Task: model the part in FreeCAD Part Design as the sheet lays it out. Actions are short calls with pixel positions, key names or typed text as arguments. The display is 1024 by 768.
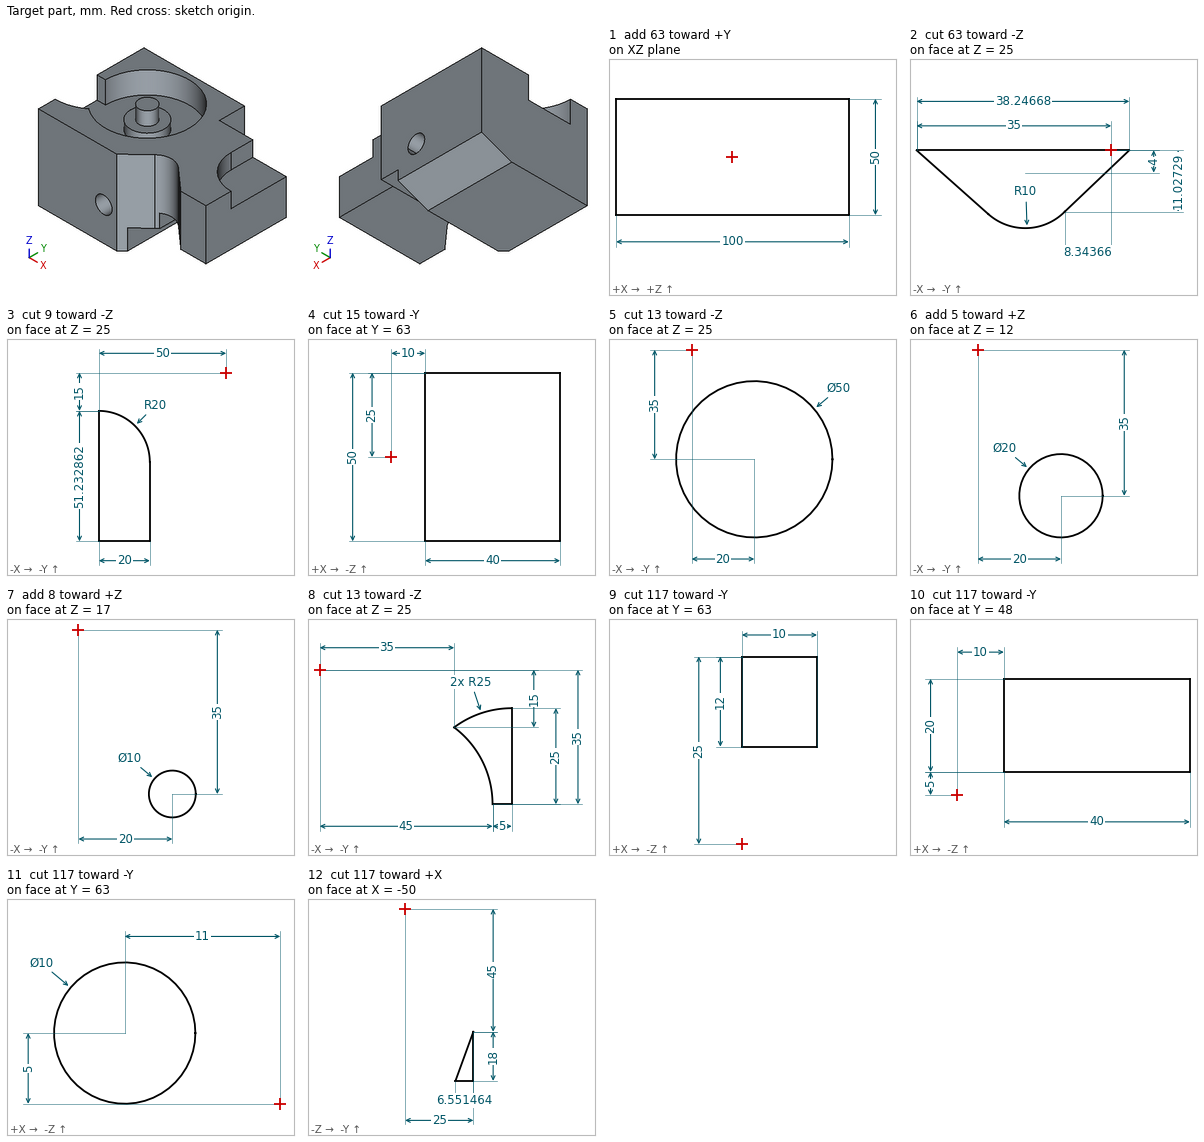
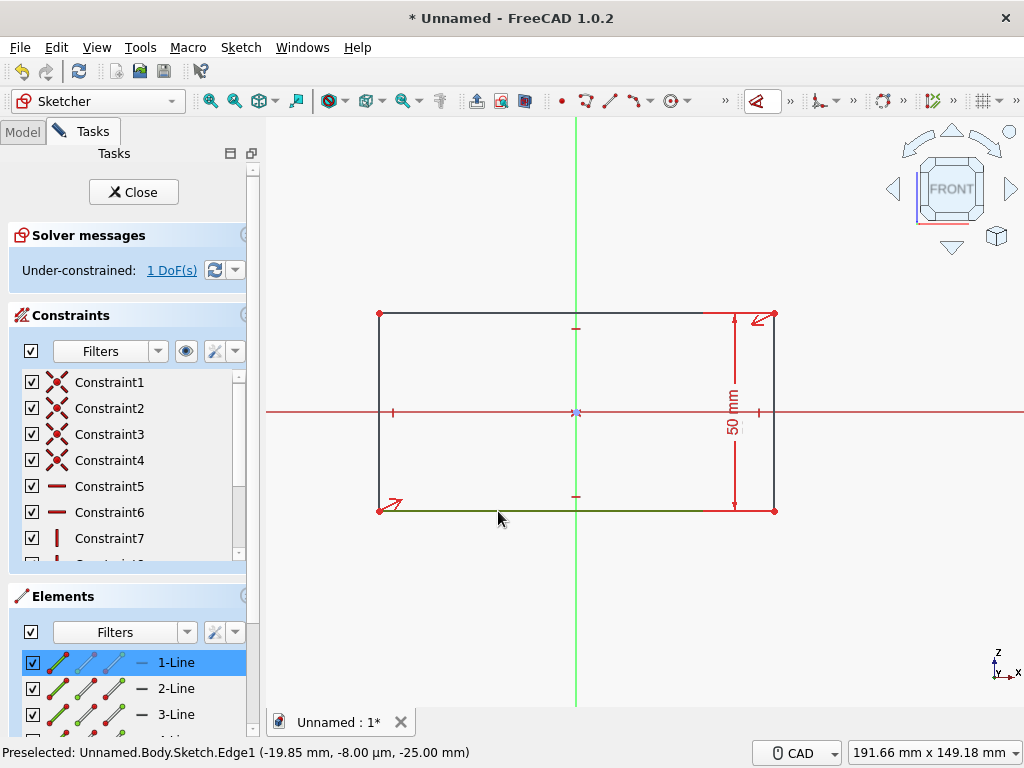
click(776, 102)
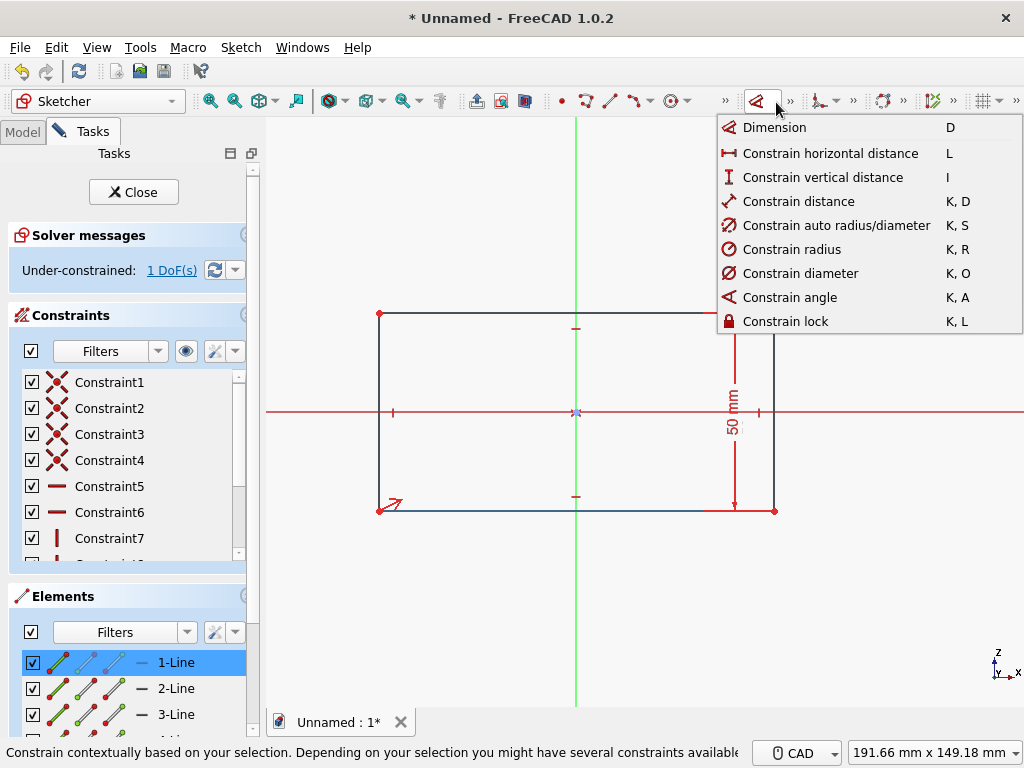
click(870, 153)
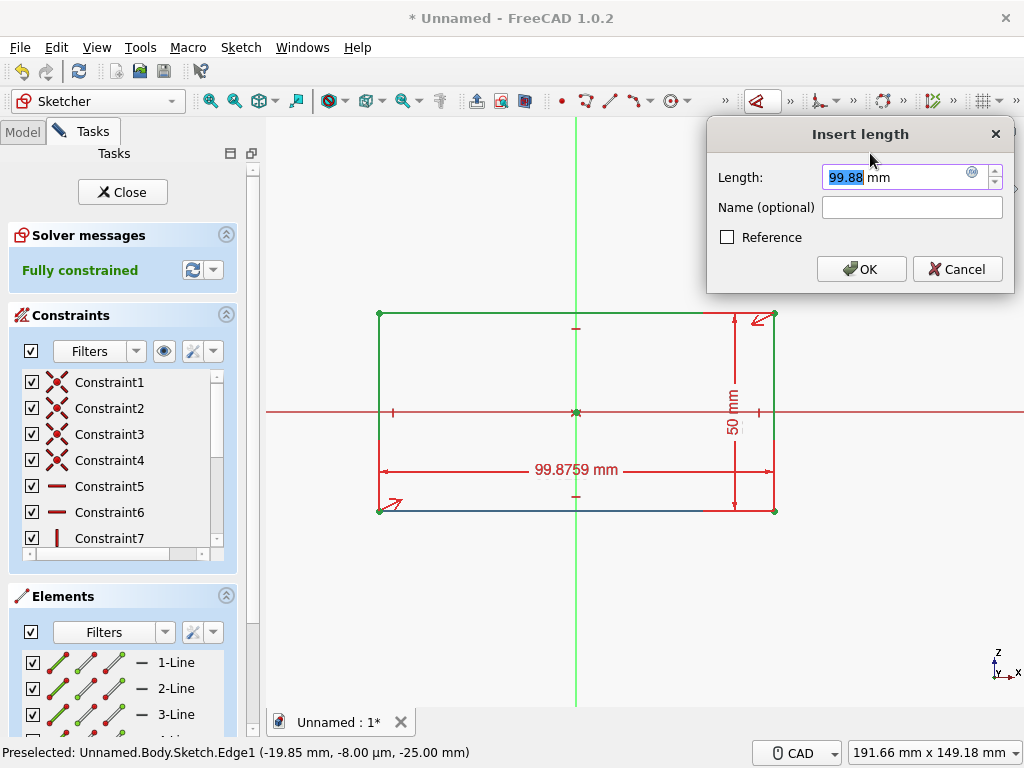
text(100)
key(Return)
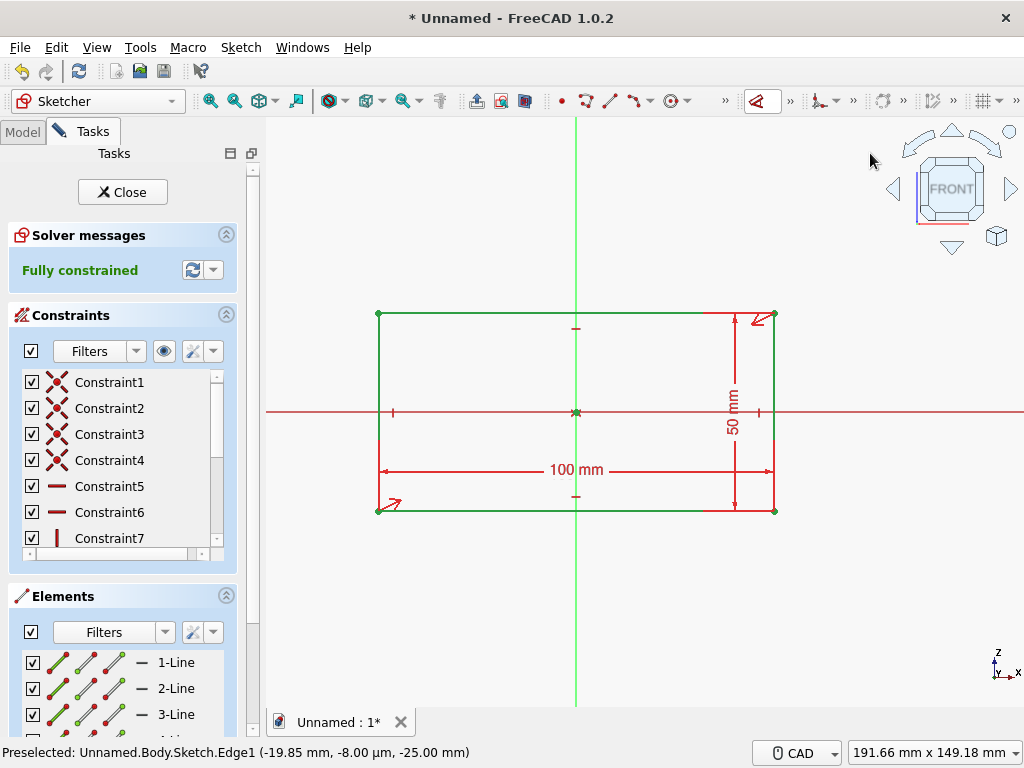
click(123, 192)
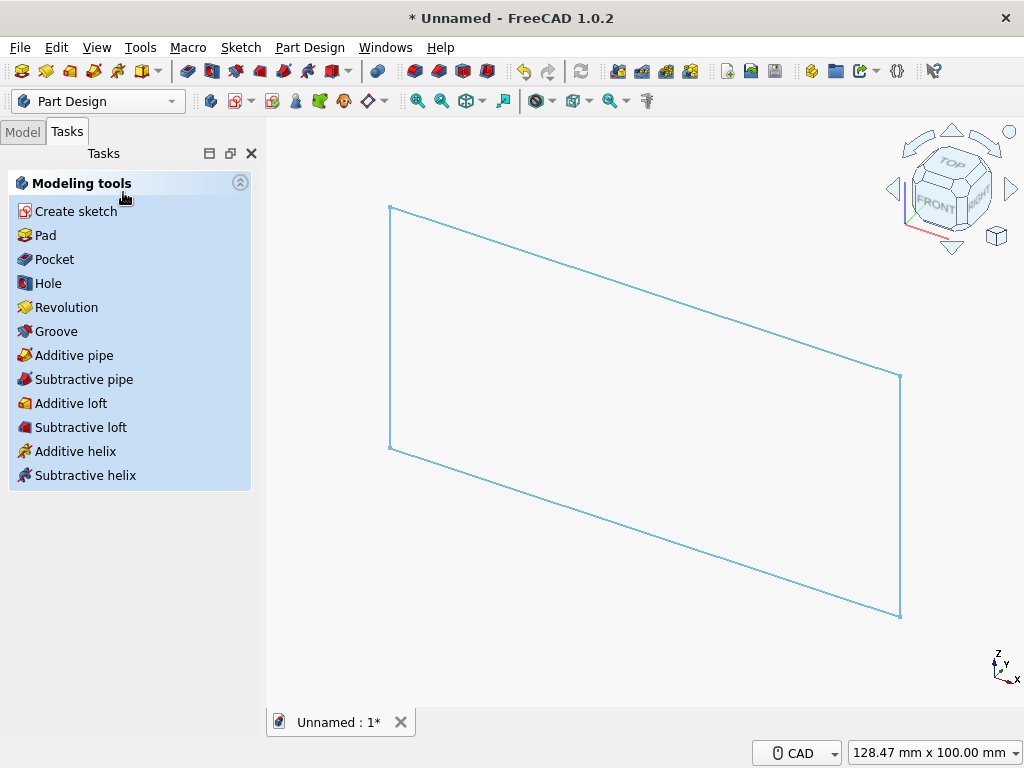
click(22, 72)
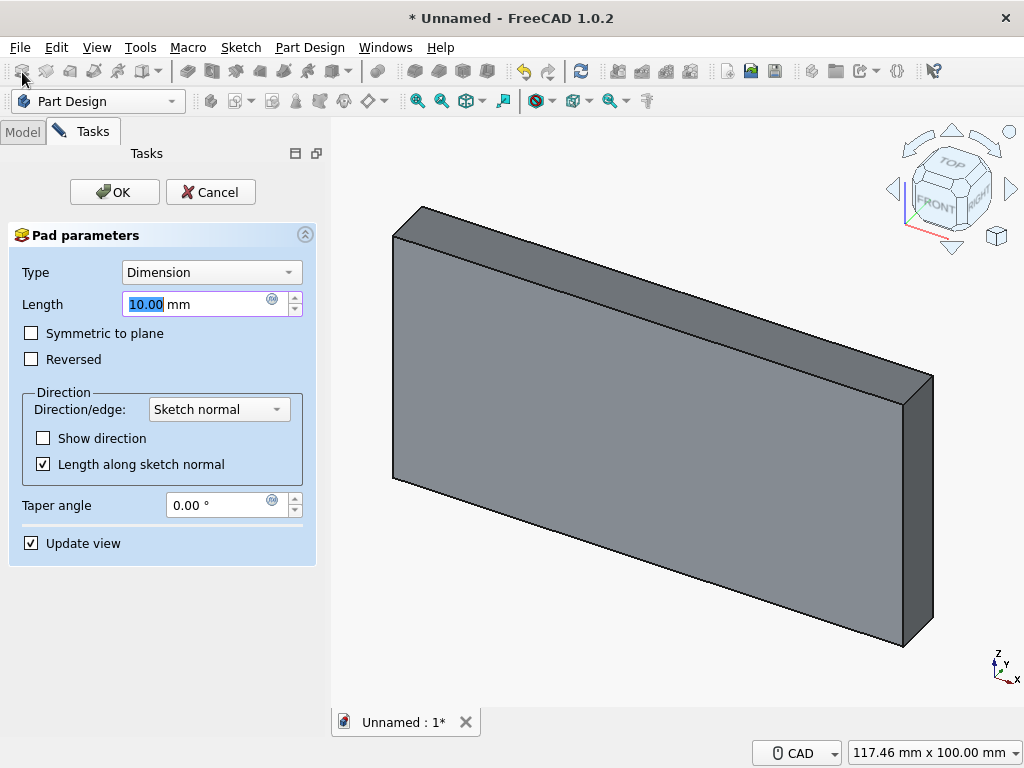
text(63)
key(Tab)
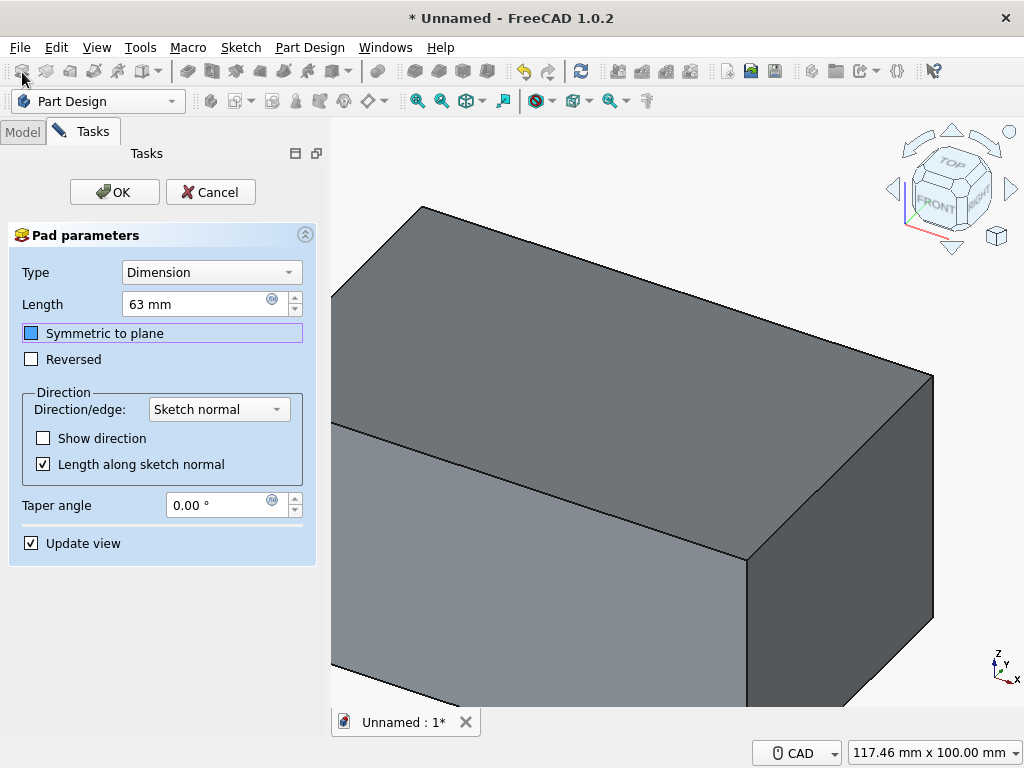
click(30, 359)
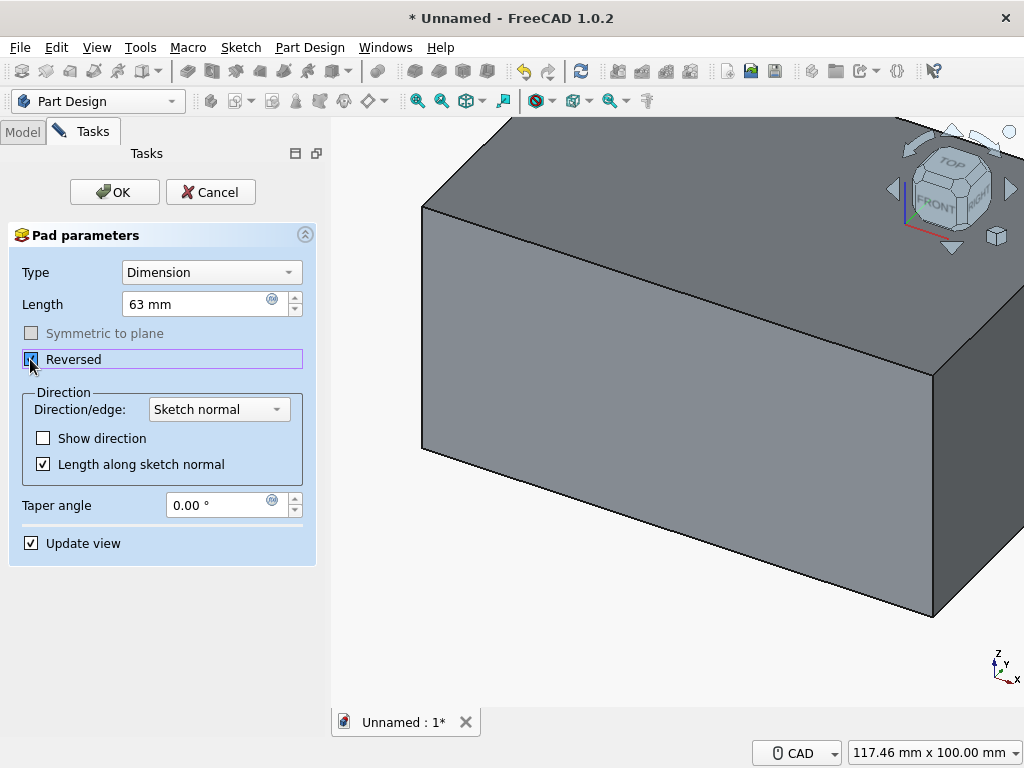
click(115, 192)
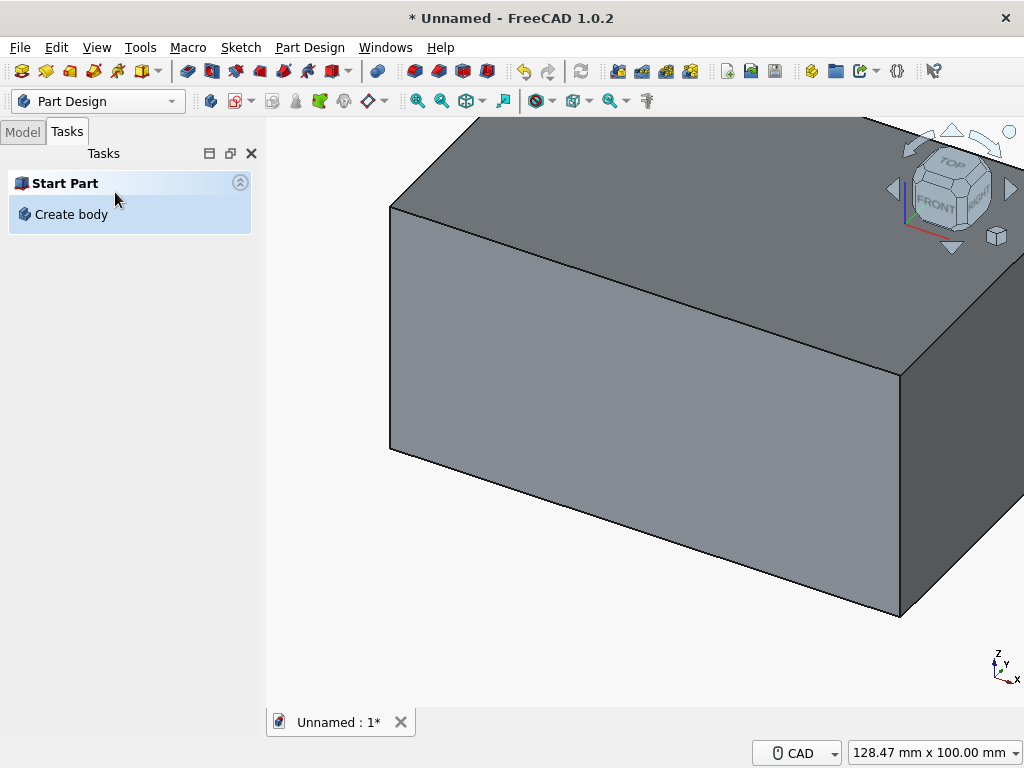
click(418, 102)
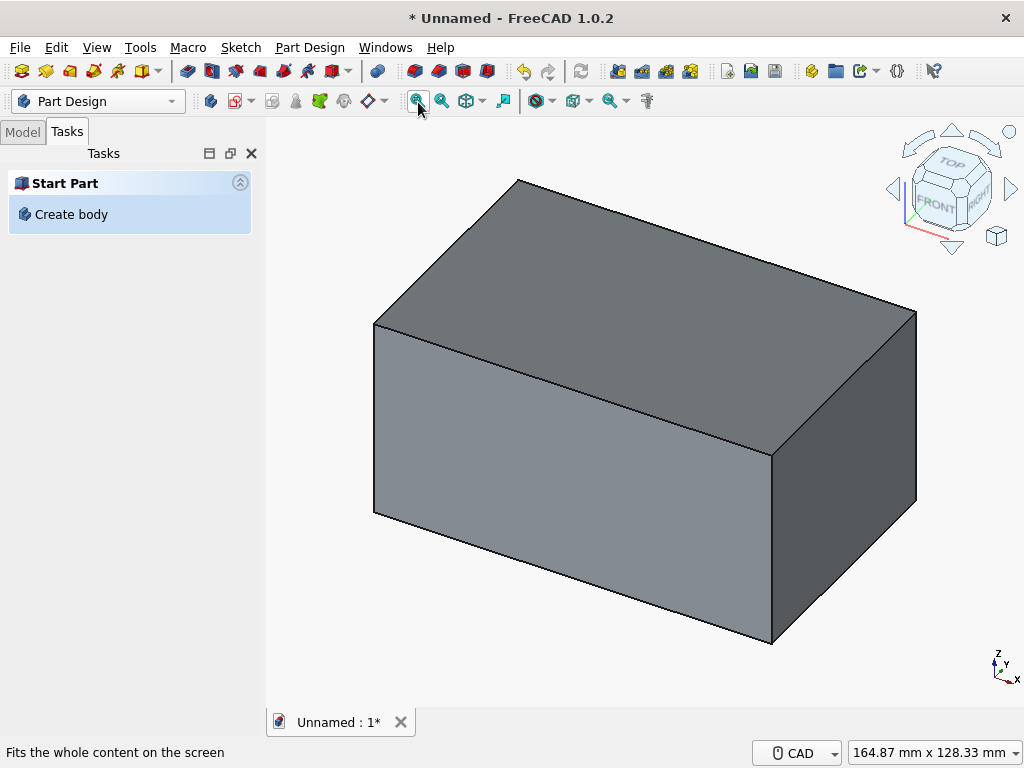
click(702, 336)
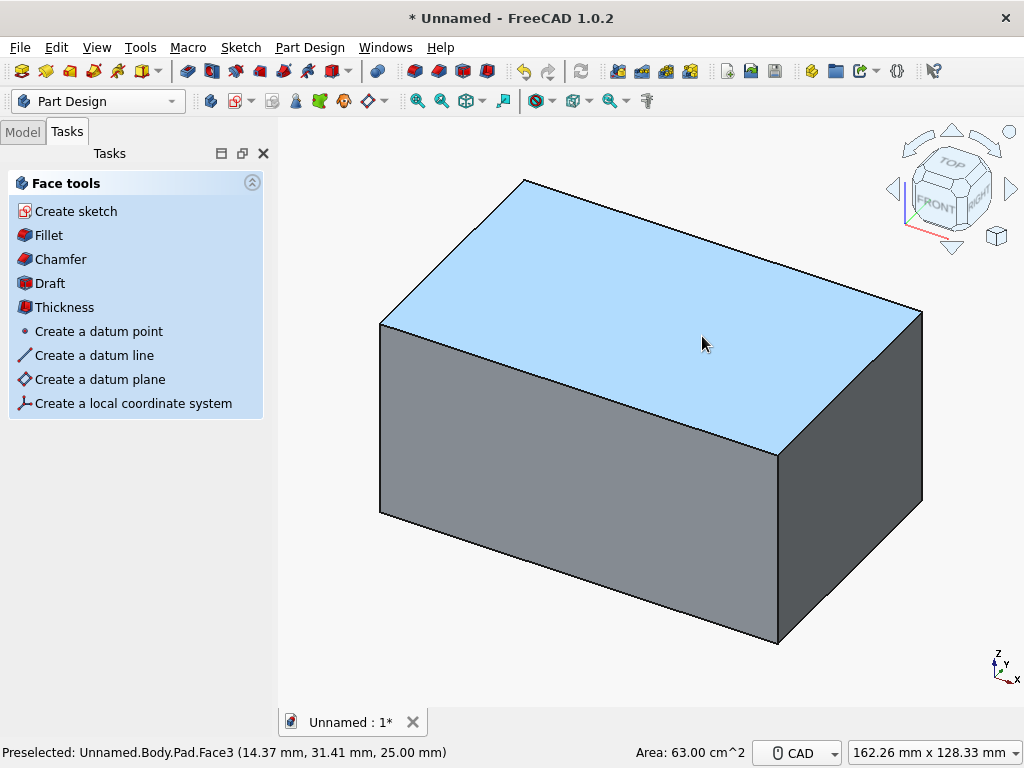
click(236, 102)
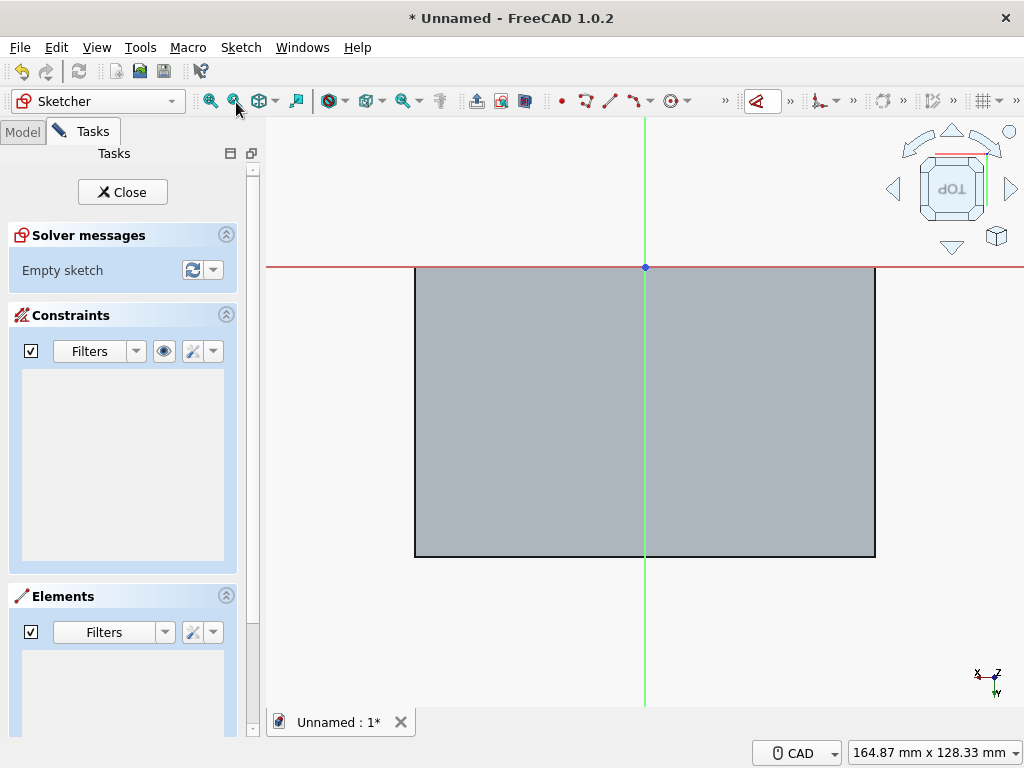
scroll(568, 207, up, 4)